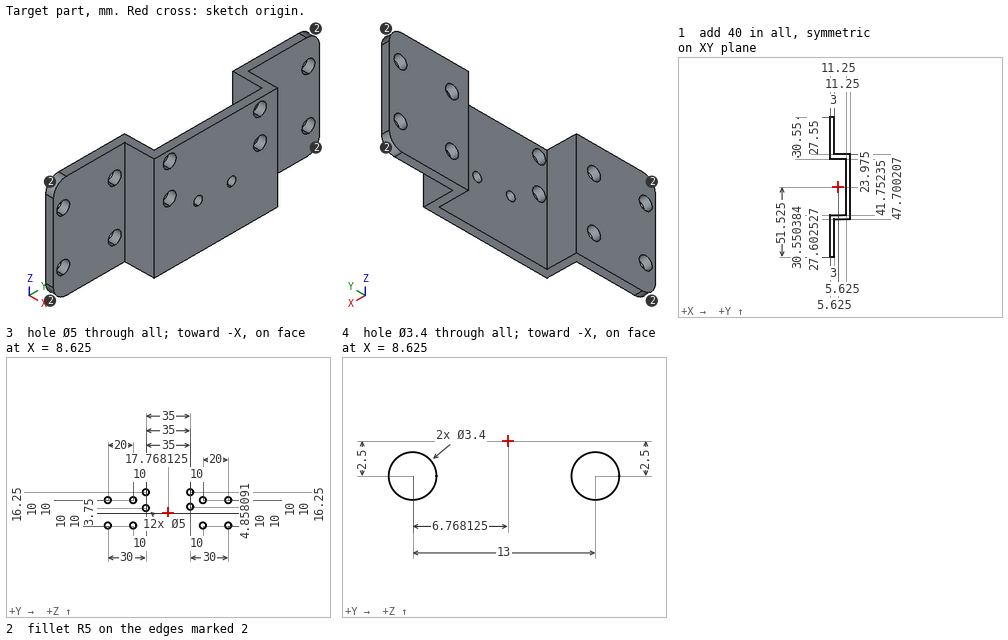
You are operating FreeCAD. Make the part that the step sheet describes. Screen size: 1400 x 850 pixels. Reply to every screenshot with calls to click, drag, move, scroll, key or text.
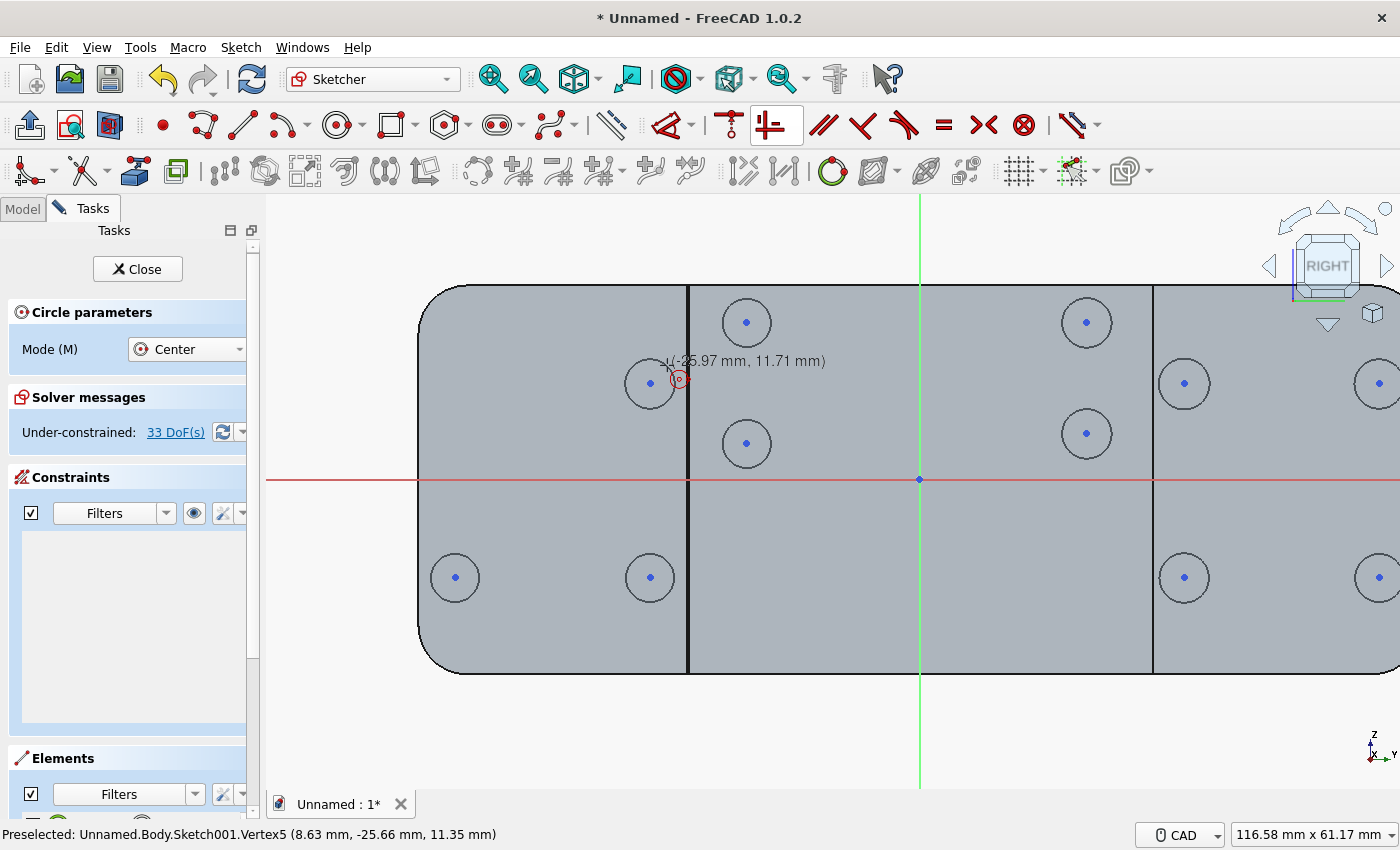
click(455, 383)
click(472, 365)
key(Escape)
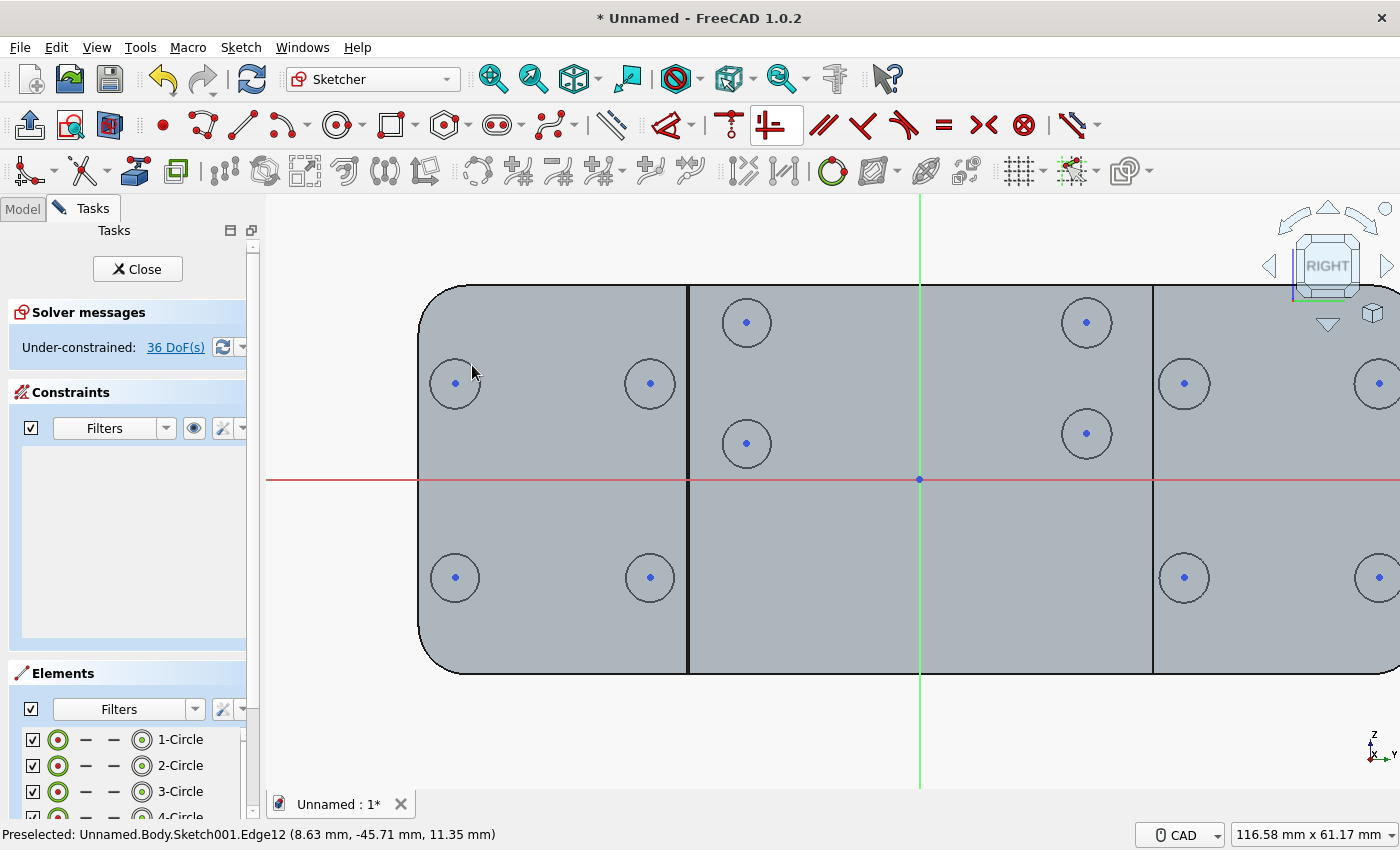
click(764, 427)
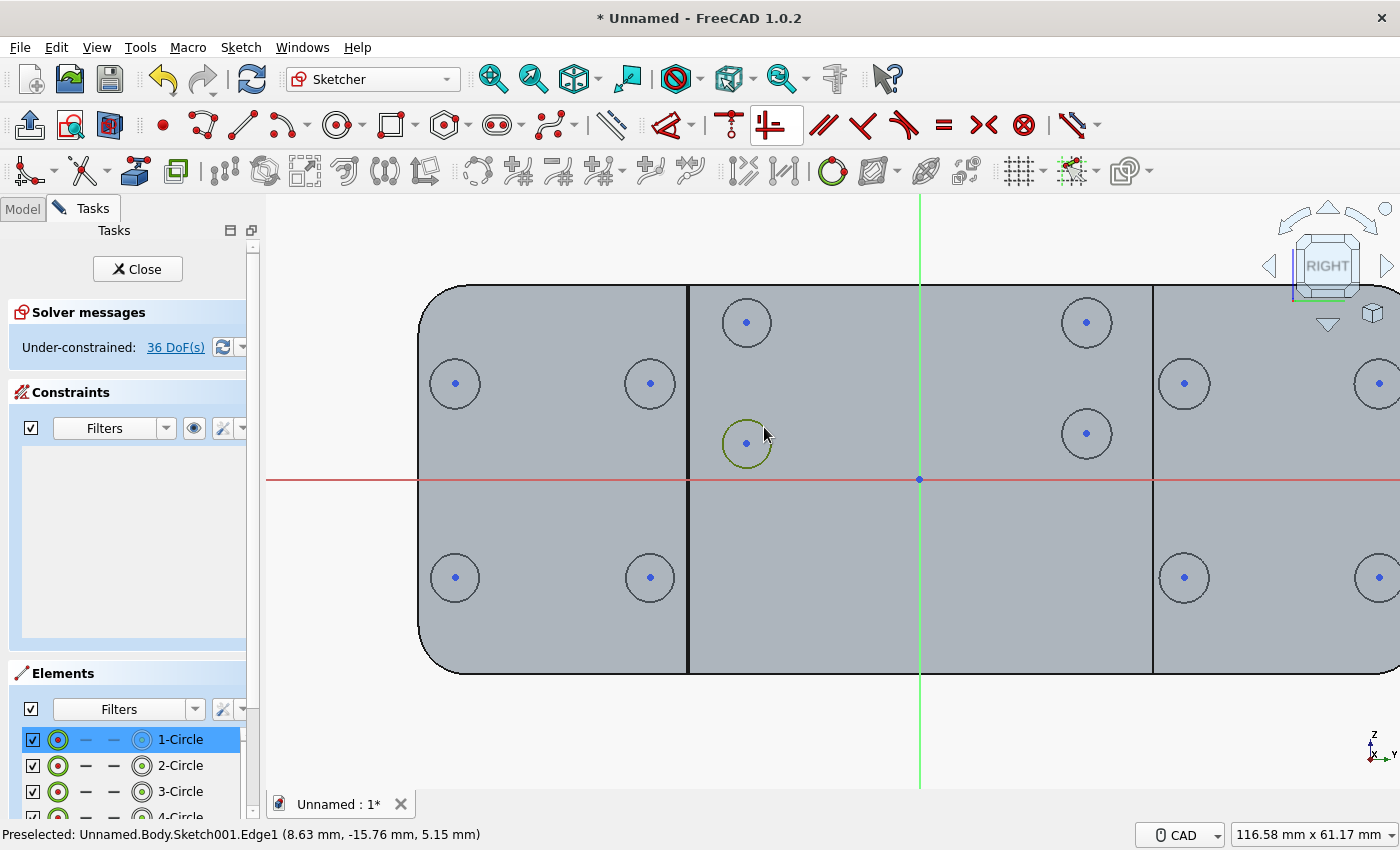
click(764, 306)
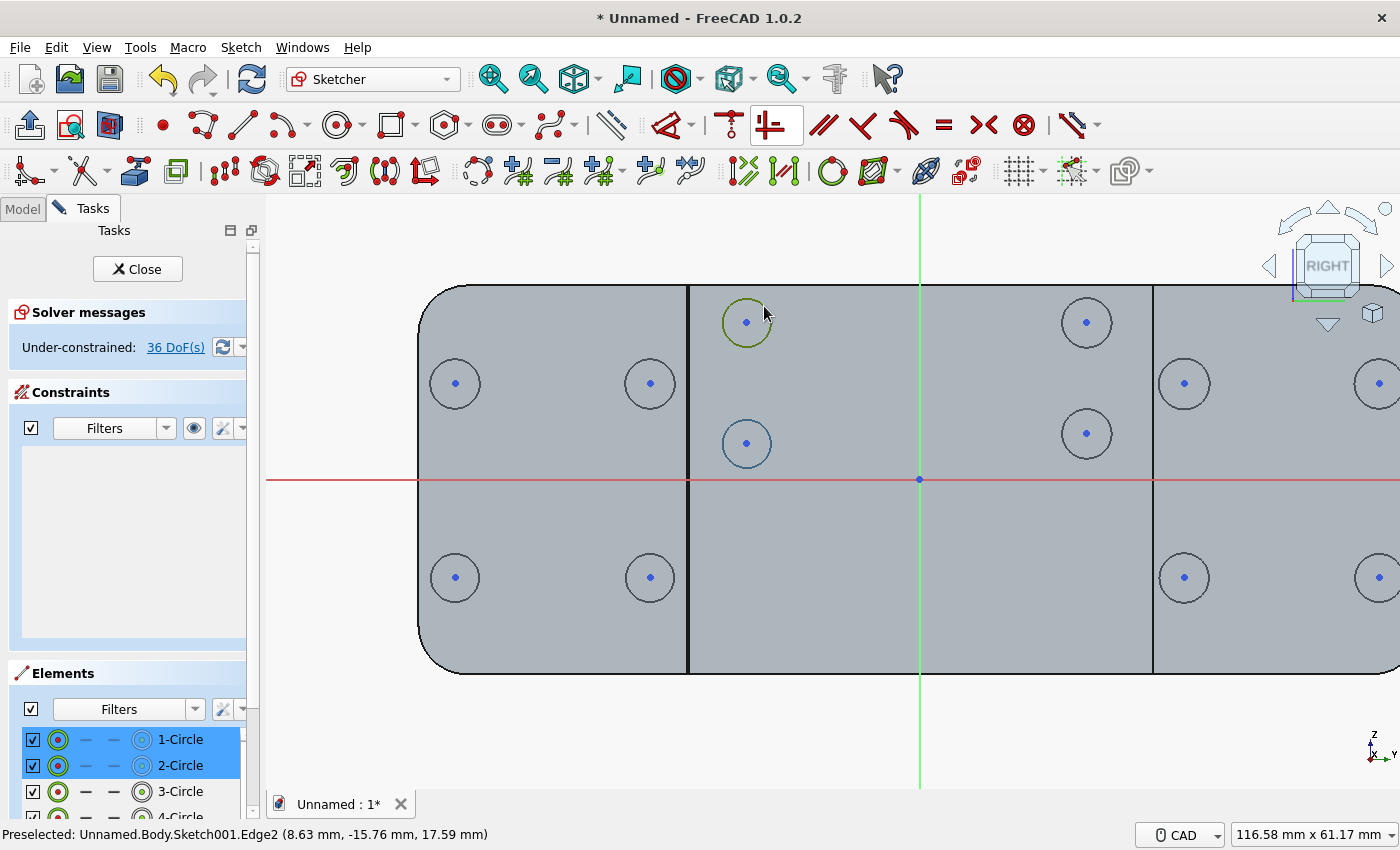
click(1104, 416)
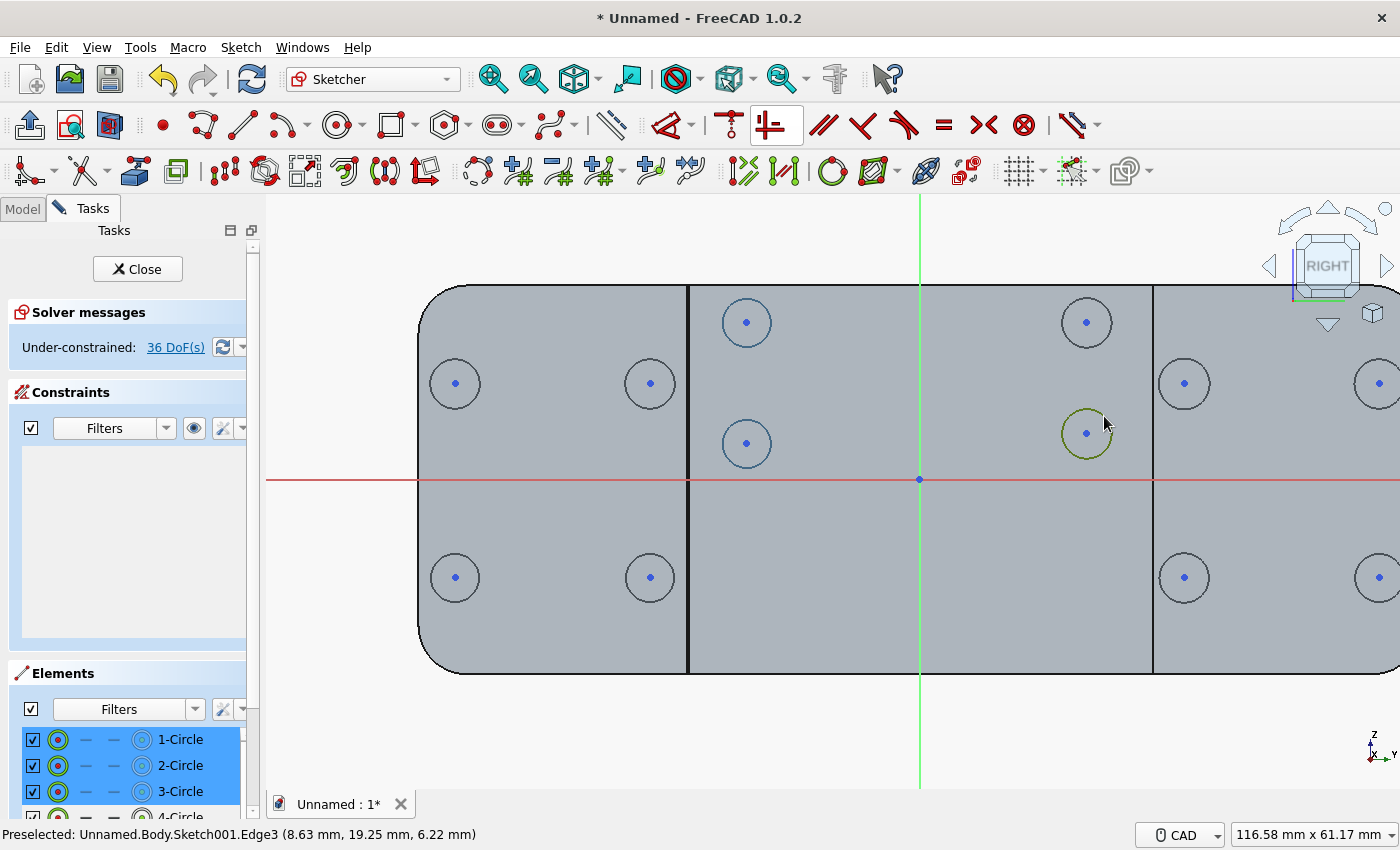
click(1104, 305)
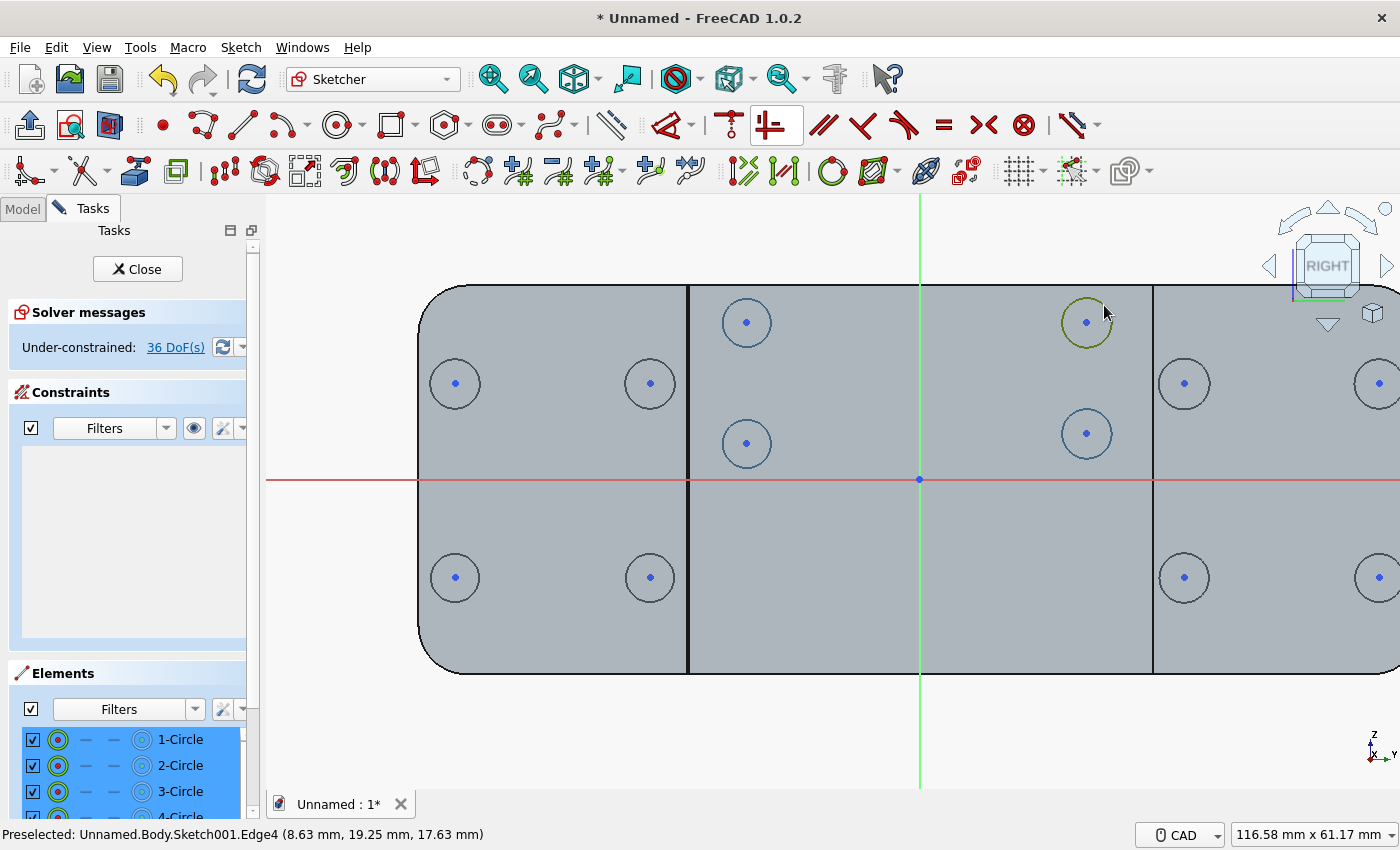
scroll(454, 577, down, 2)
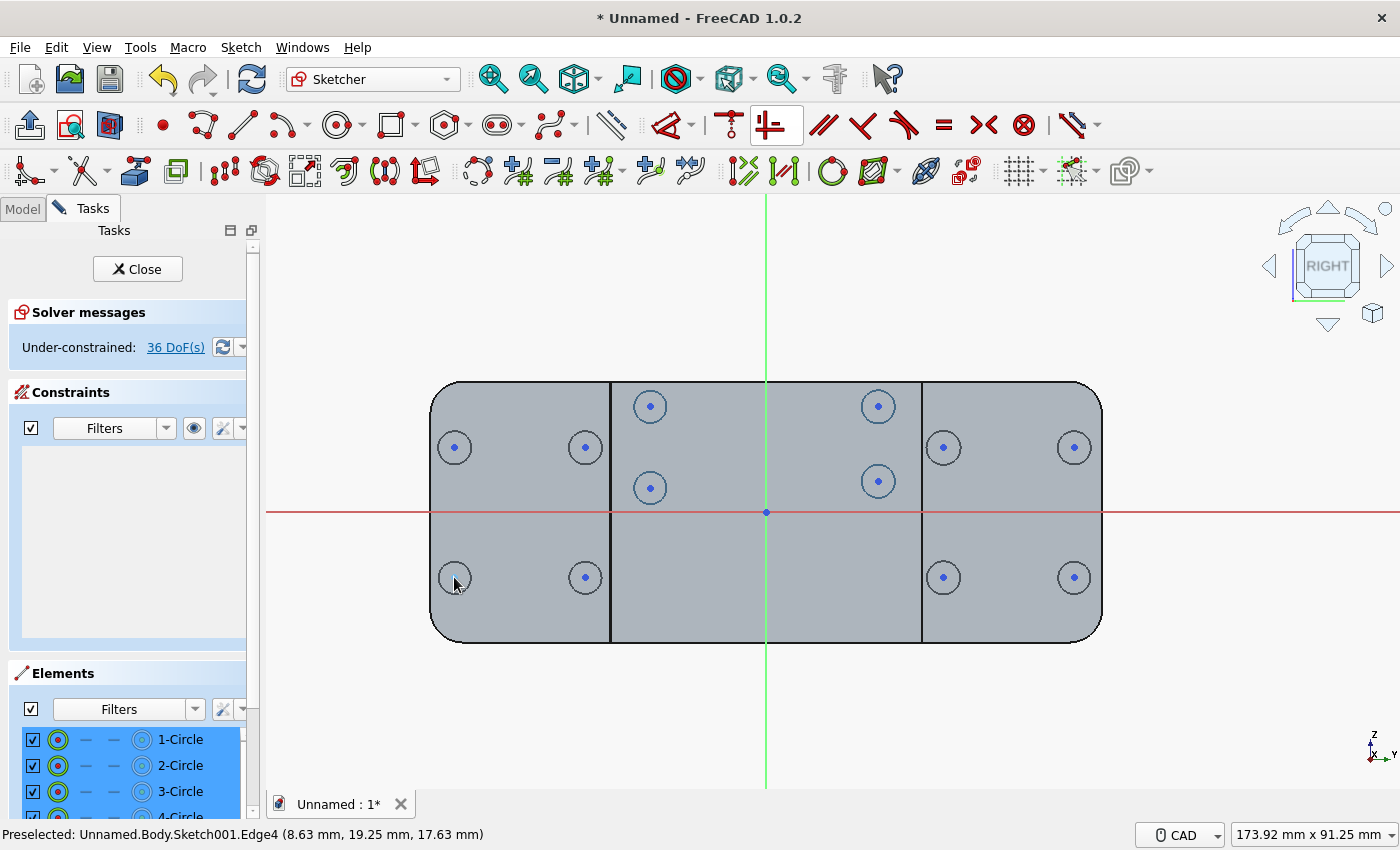
click(1086, 566)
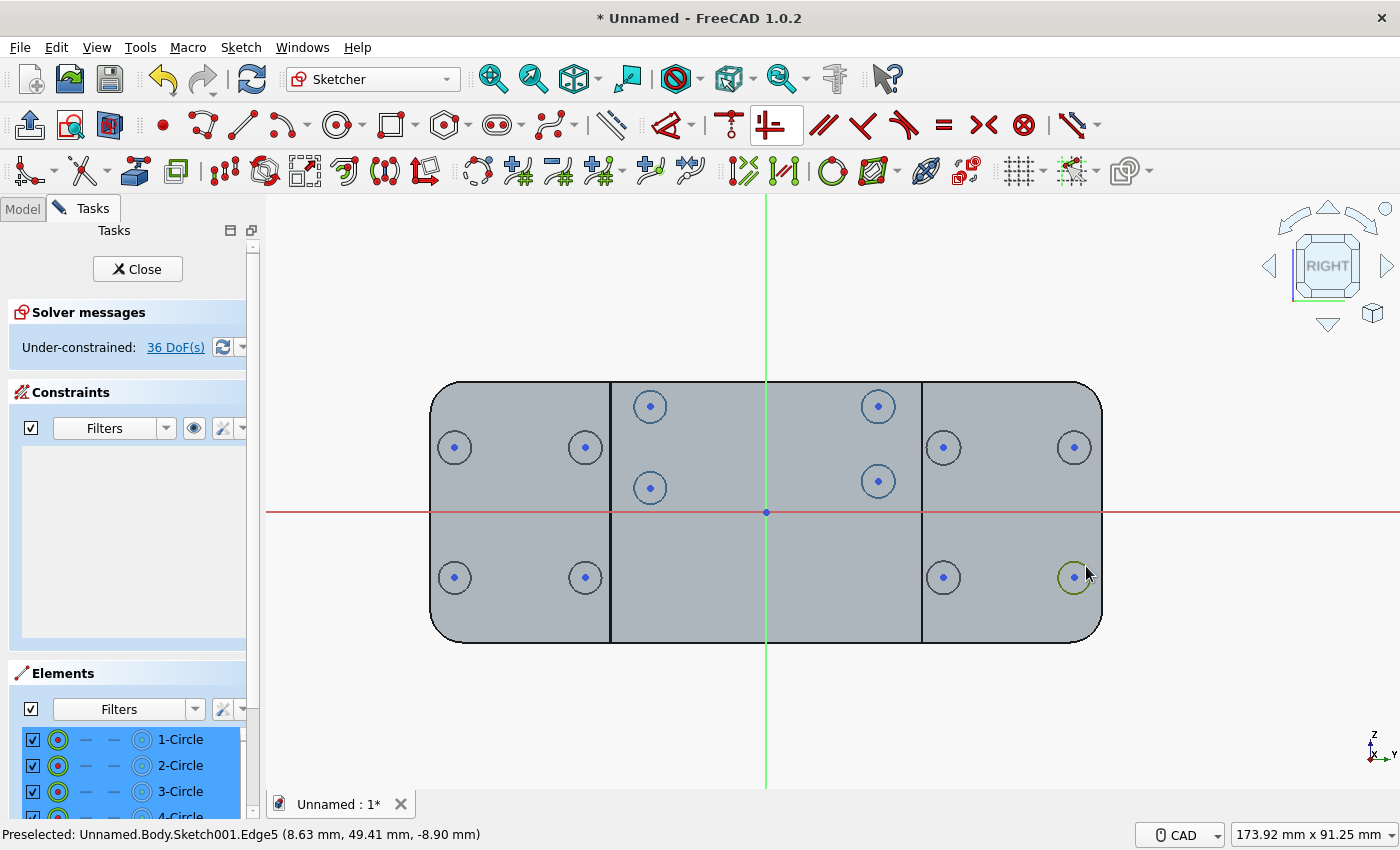
click(955, 566)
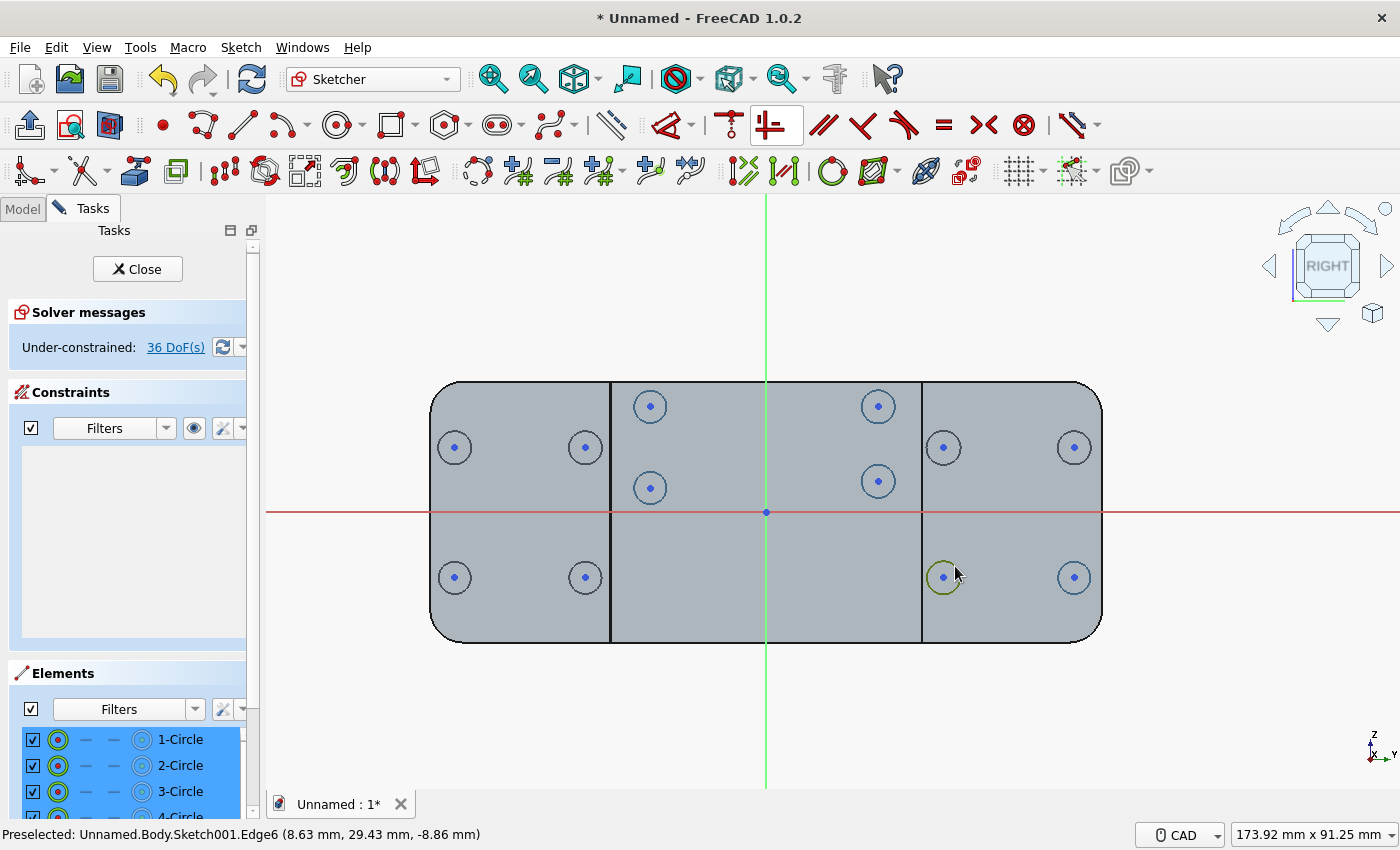
click(956, 436)